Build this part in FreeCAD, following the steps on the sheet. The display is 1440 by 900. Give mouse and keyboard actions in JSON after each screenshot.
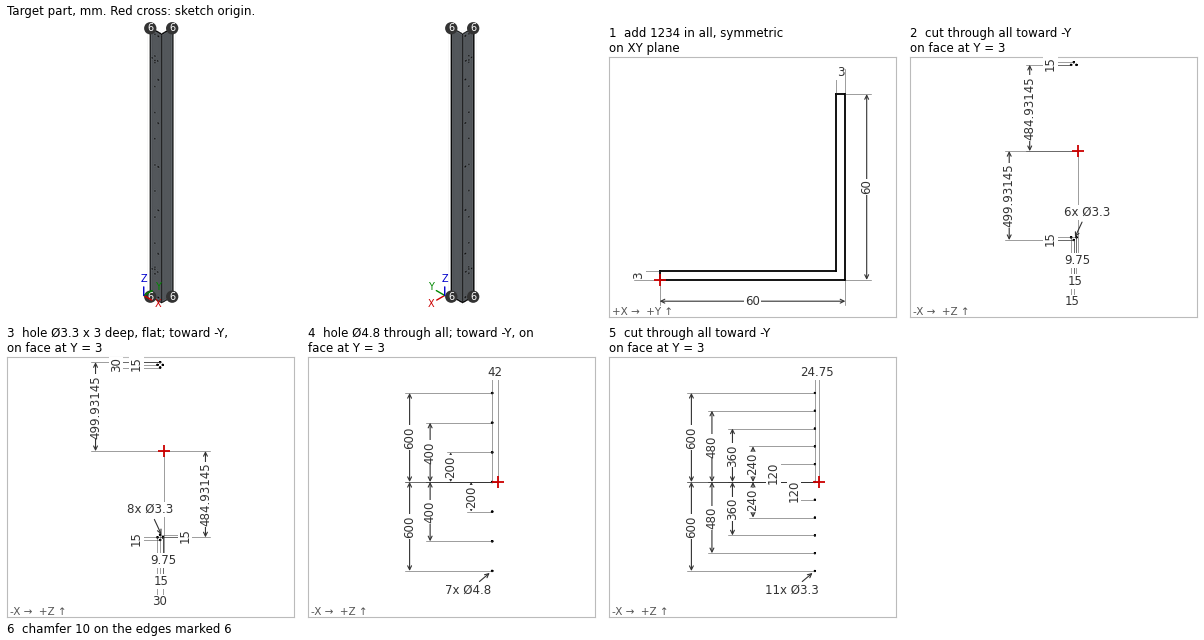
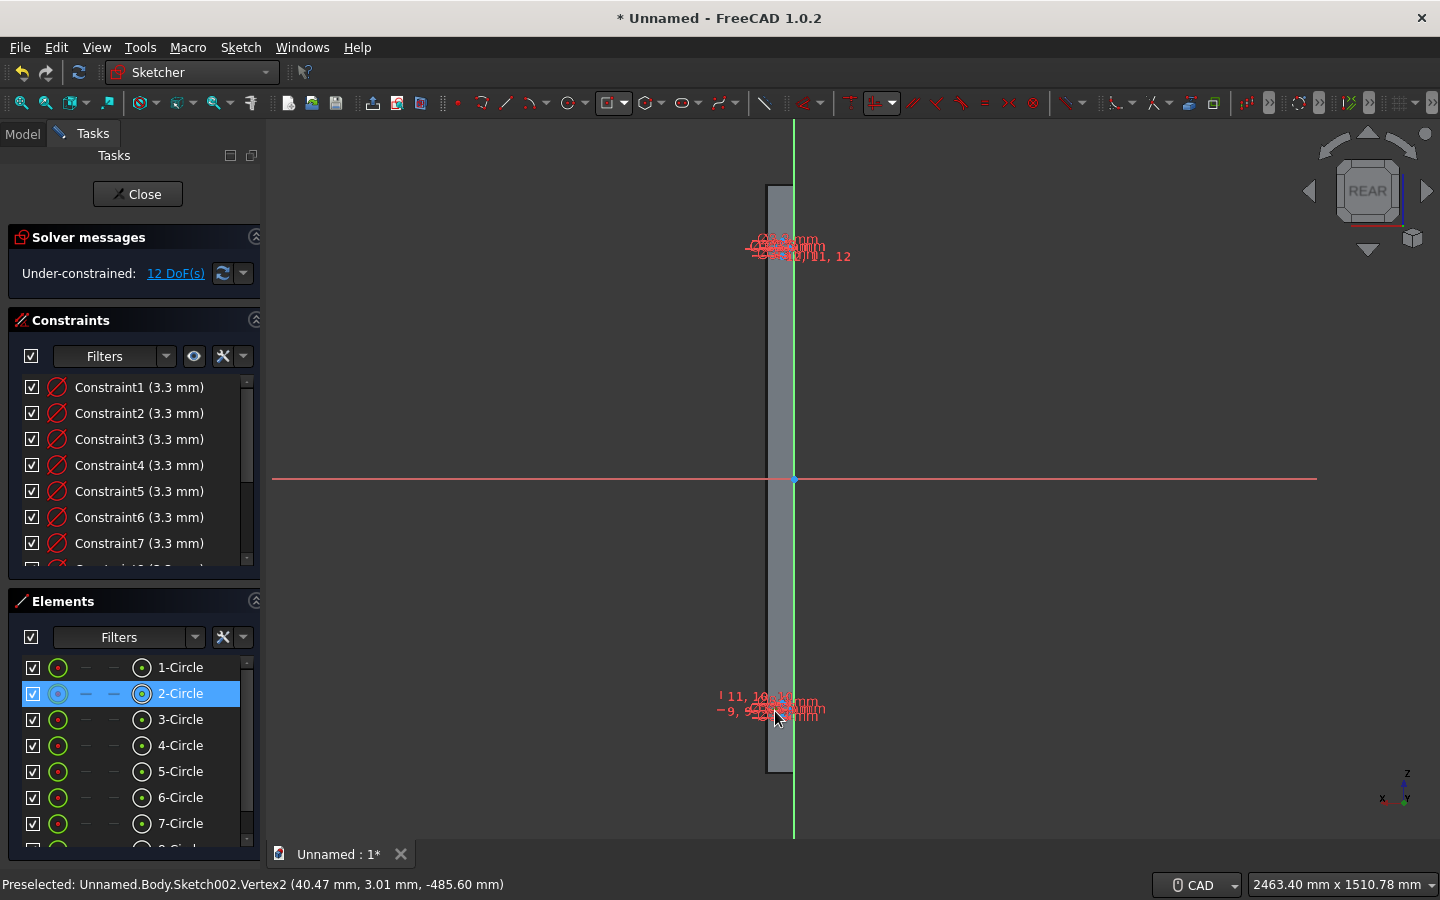
{"action": "left_click", "coordinate": [773, 247]}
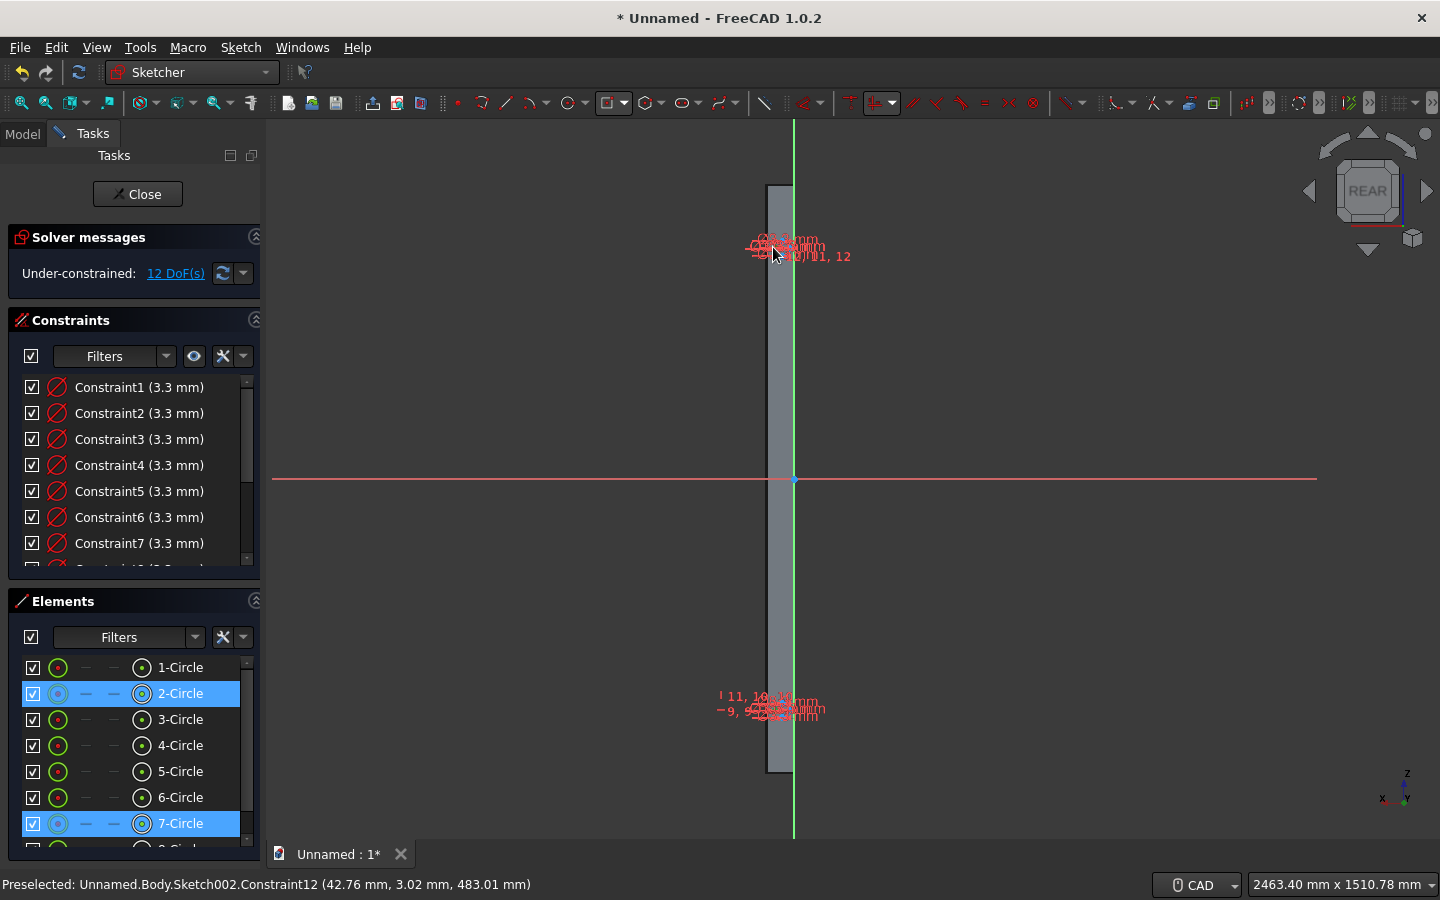
{"action": "key", "text": "v"}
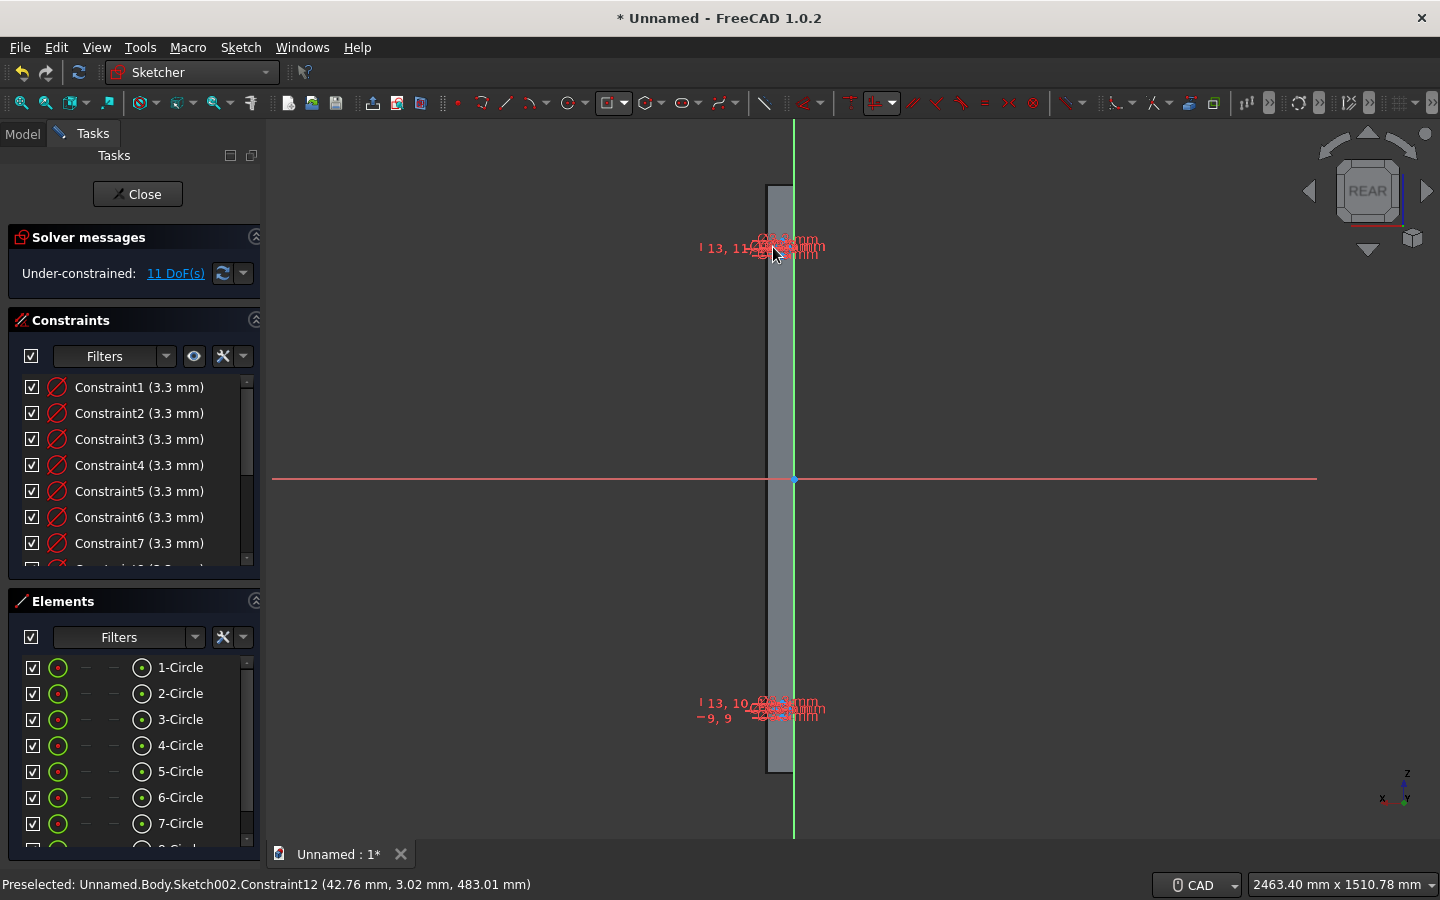
{"action": "left_click", "coordinate": [790, 711]}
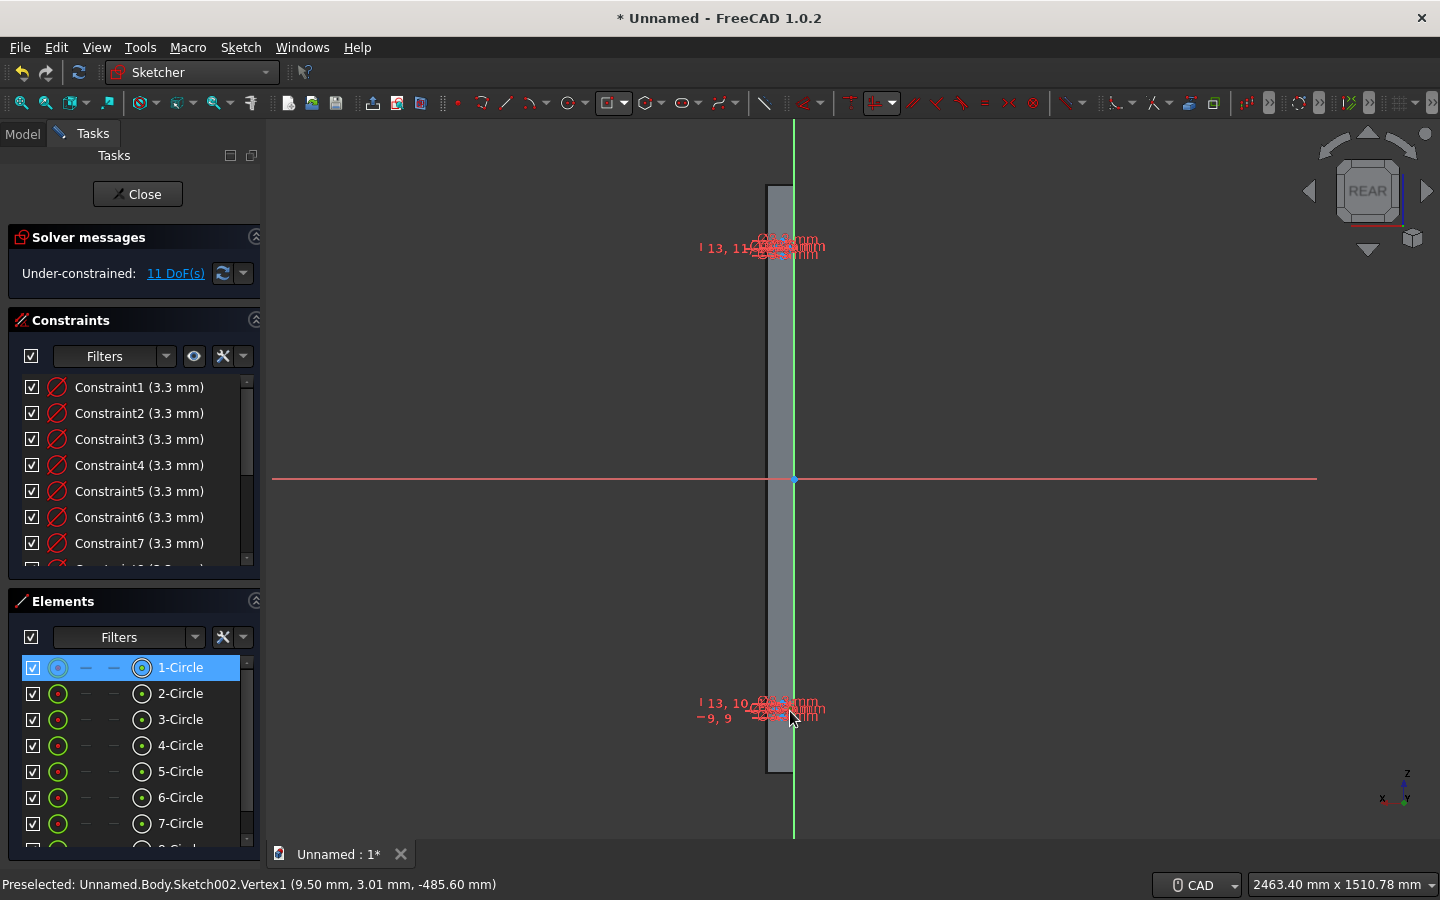
{"action": "scroll", "coordinate": [790, 248], "scroll_direction": "up", "scroll_amount": 2}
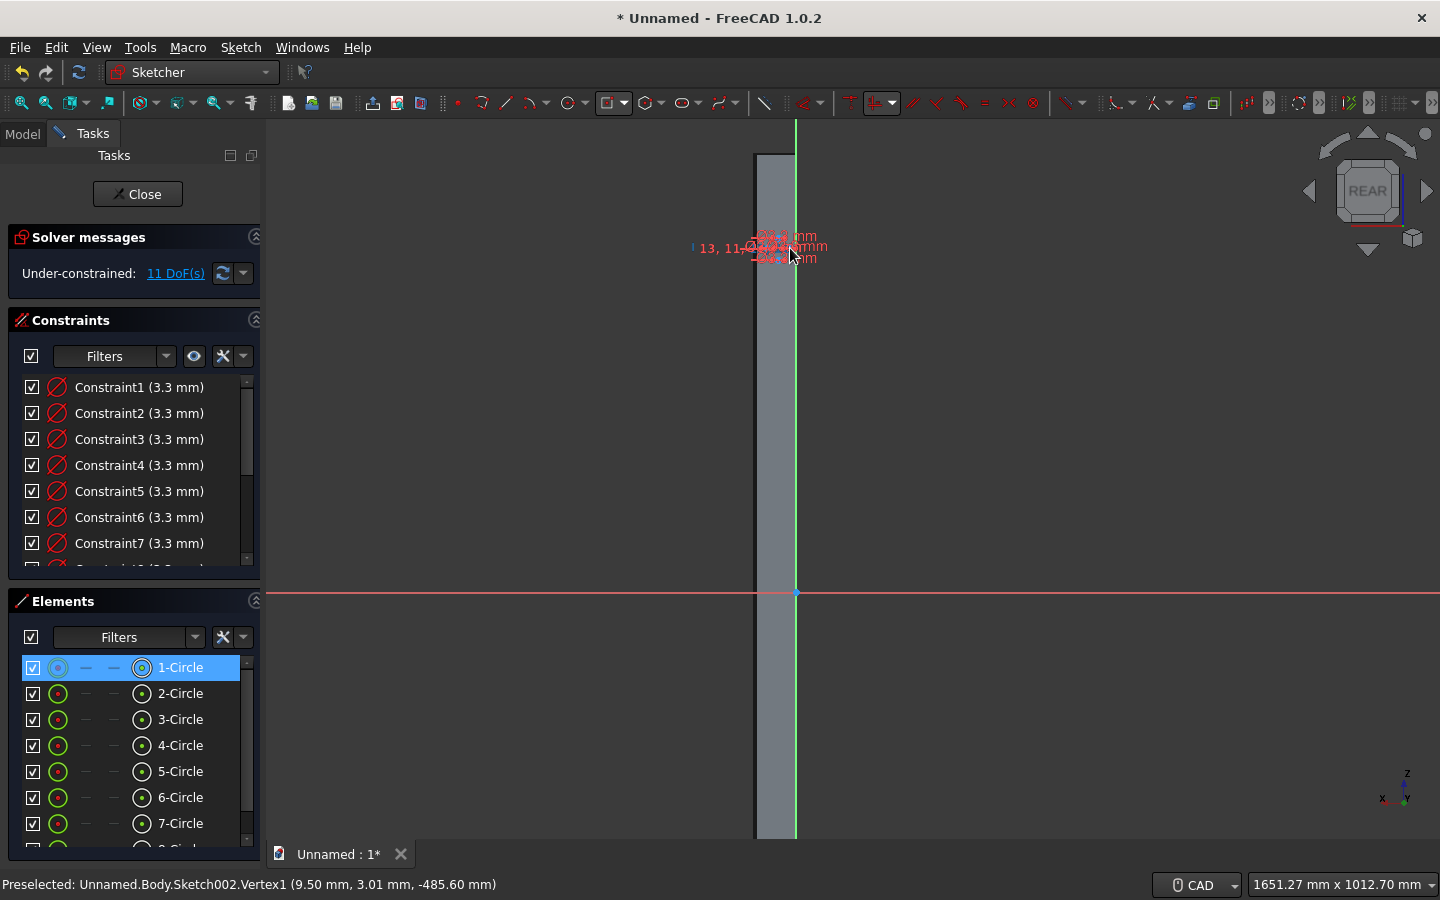
{"action": "left_click", "coordinate": [791, 250]}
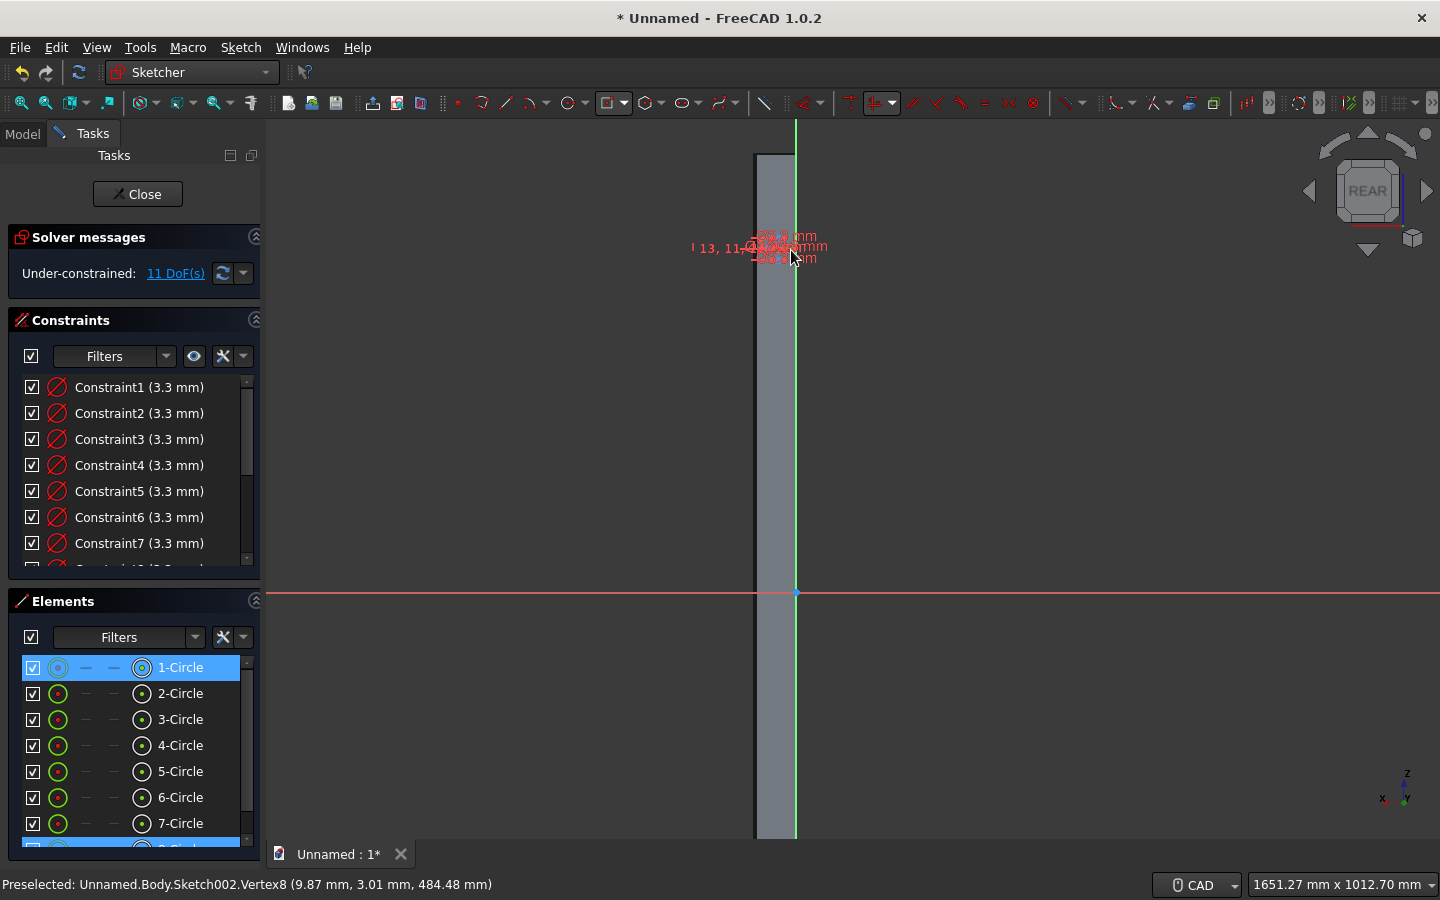
{"action": "left_click", "coordinate": [894, 104]}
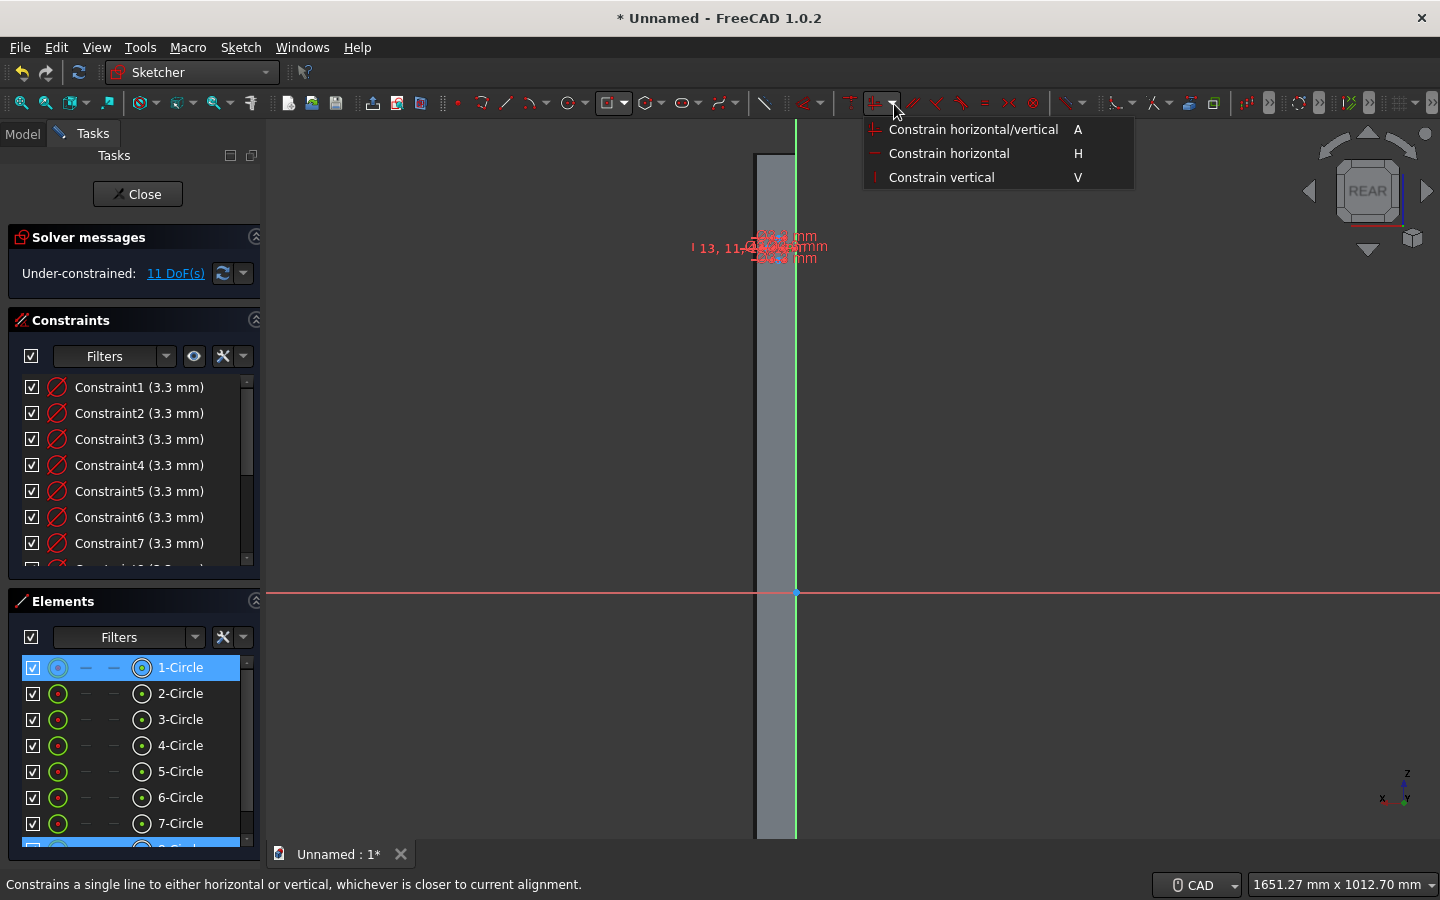
{"action": "left_click", "coordinate": [999, 177]}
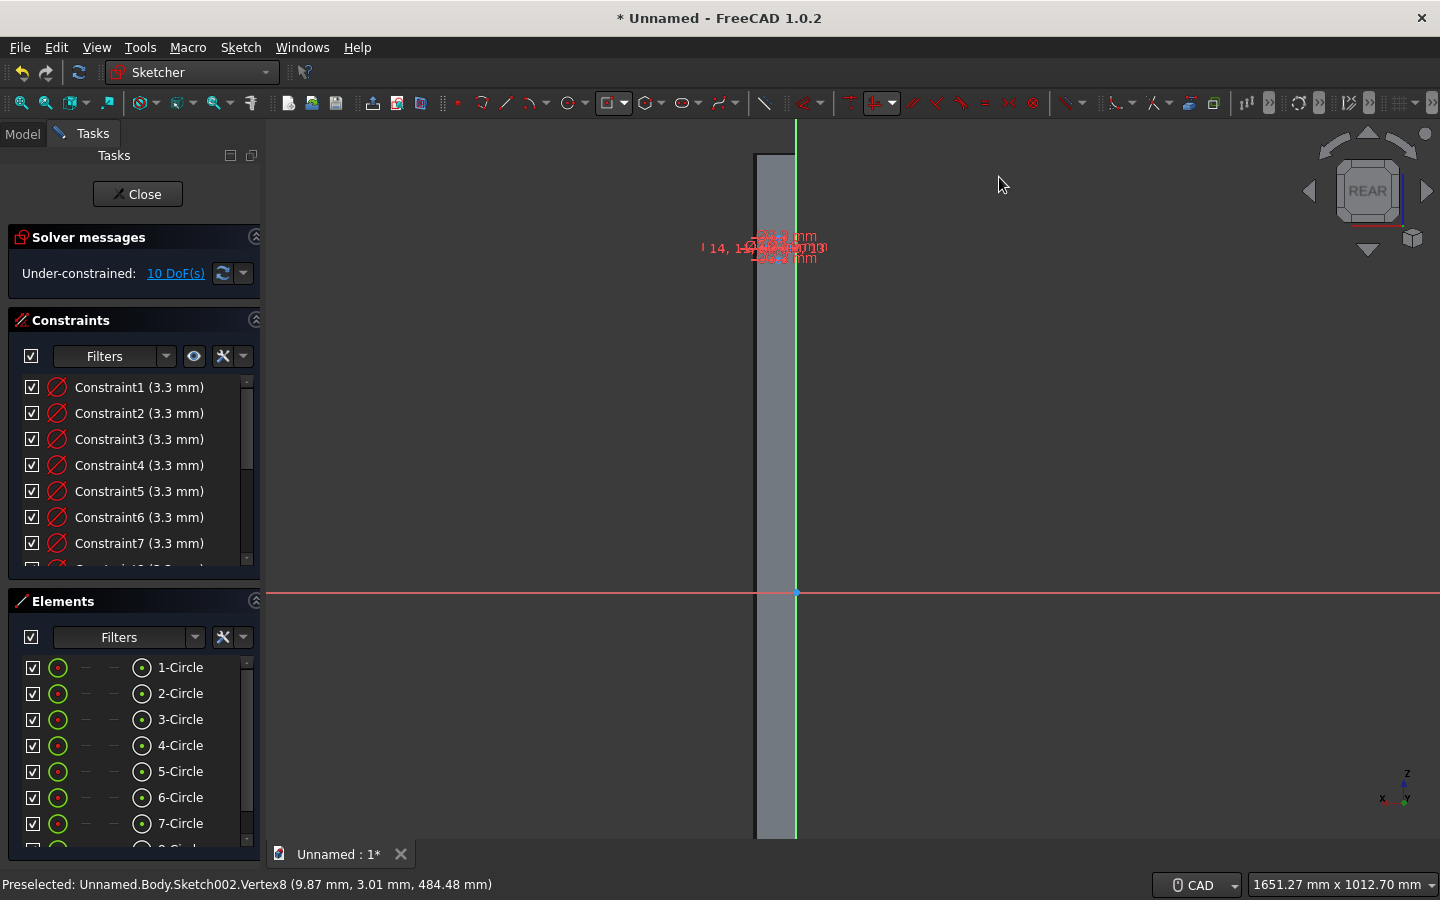
{"action": "scroll", "coordinate": [768, 249], "scroll_direction": "up", "scroll_amount": 4}